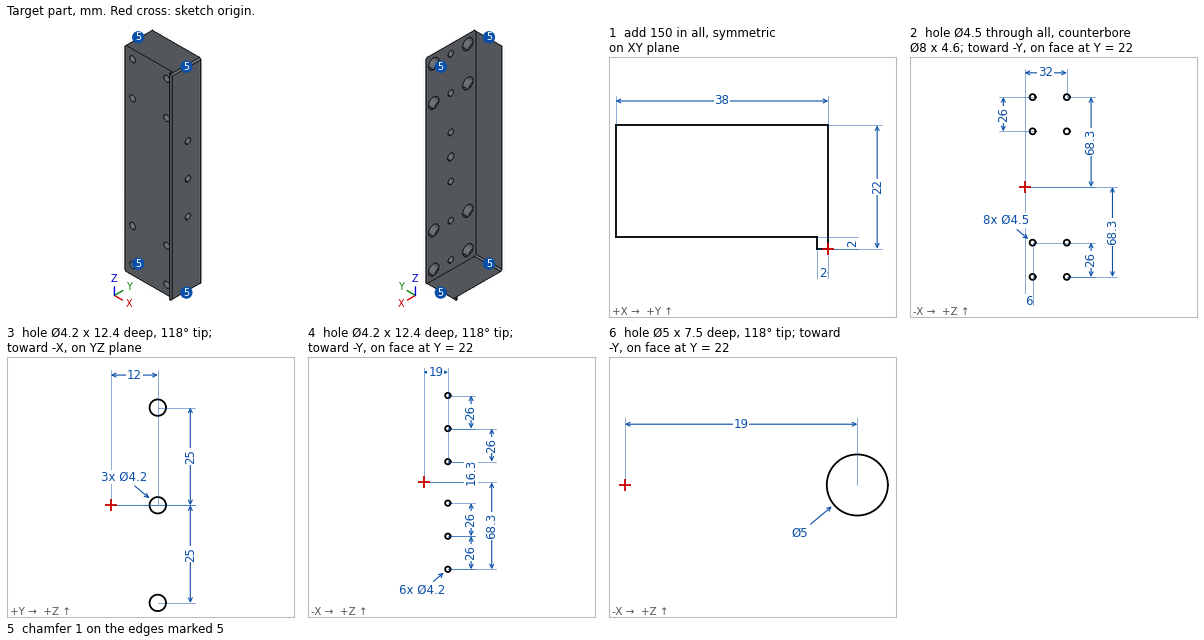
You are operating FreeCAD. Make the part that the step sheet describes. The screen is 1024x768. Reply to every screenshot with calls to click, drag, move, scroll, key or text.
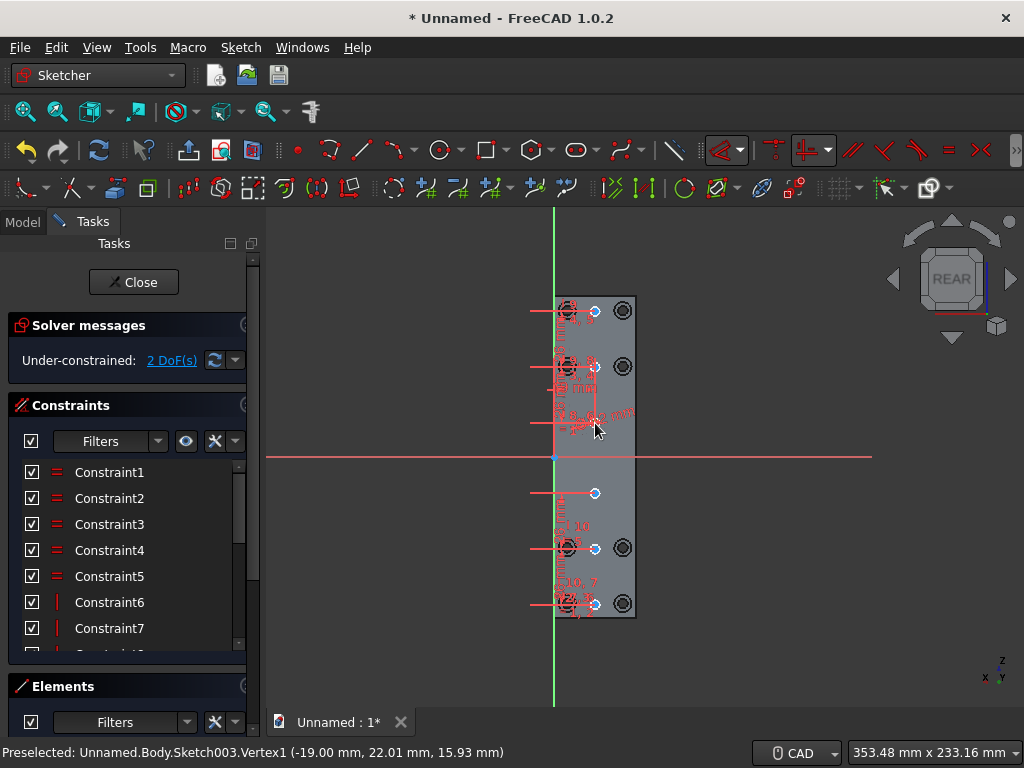
key(i)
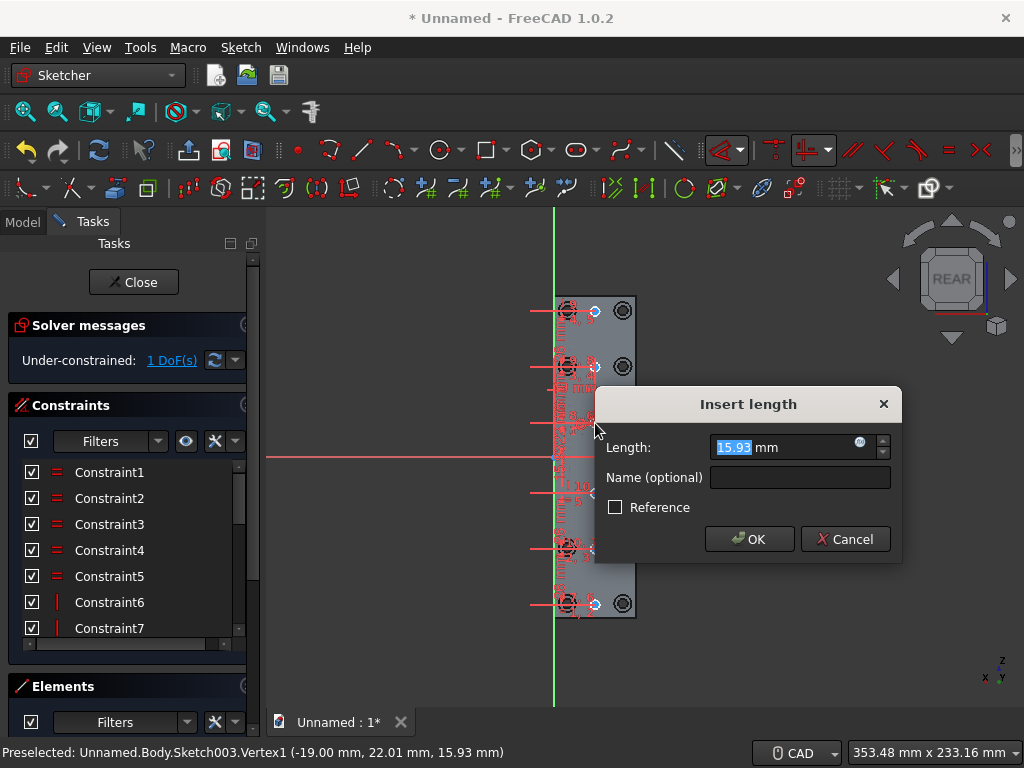
text(16.3)
key(Return)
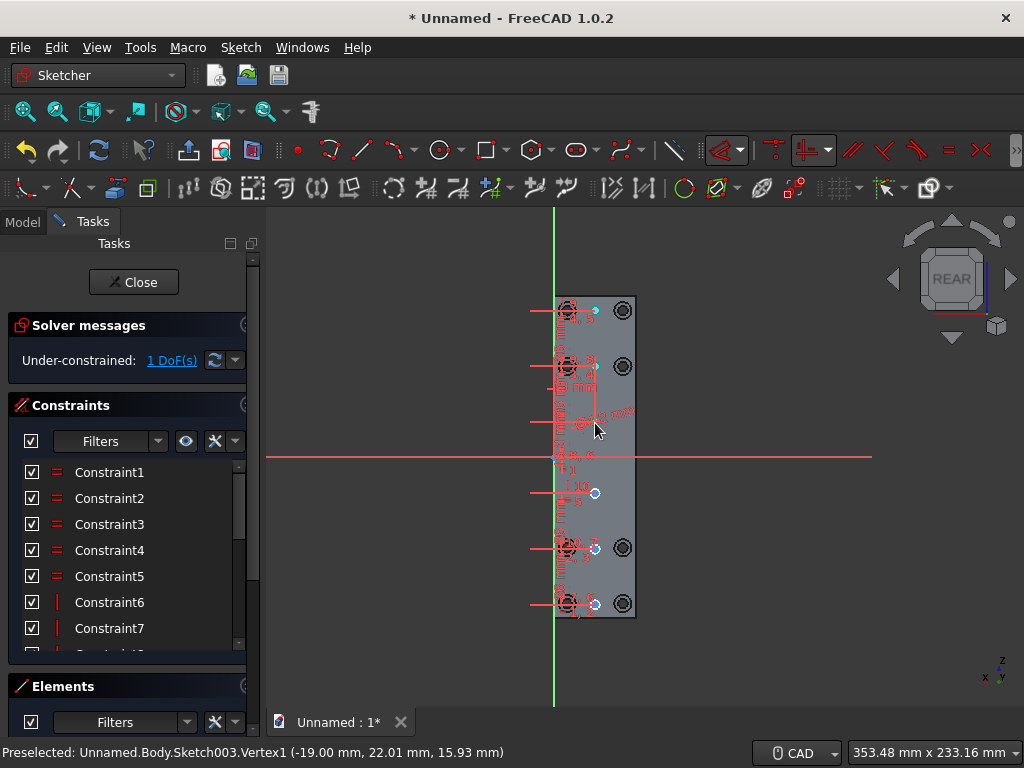
click(595, 605)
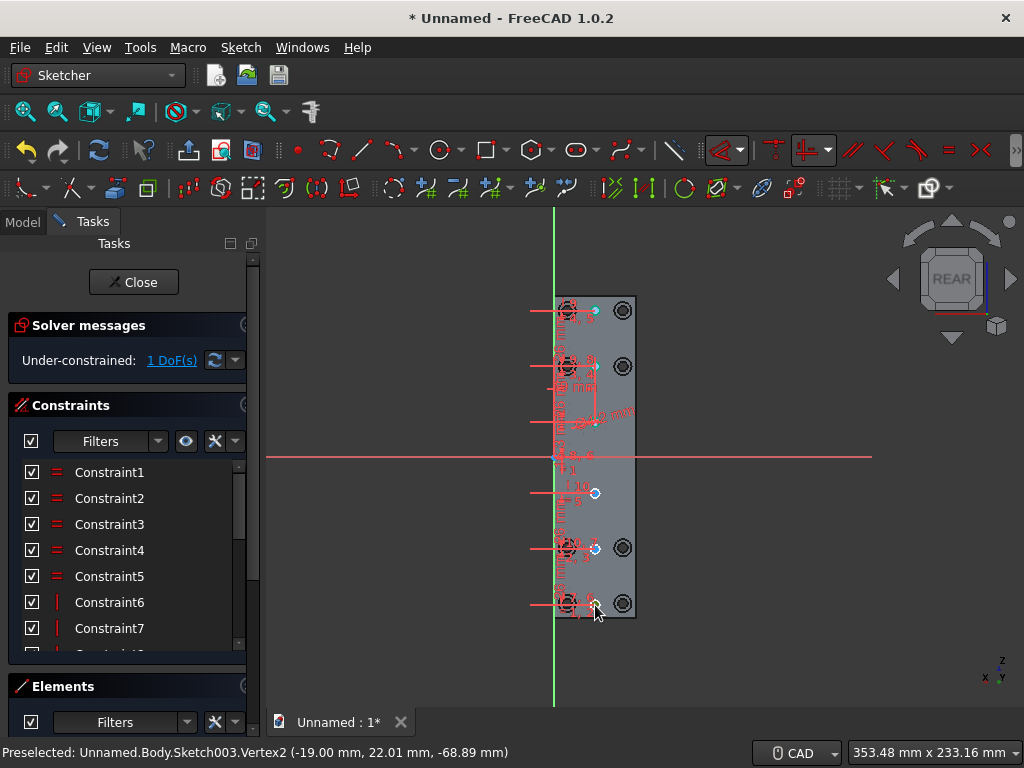
key(i)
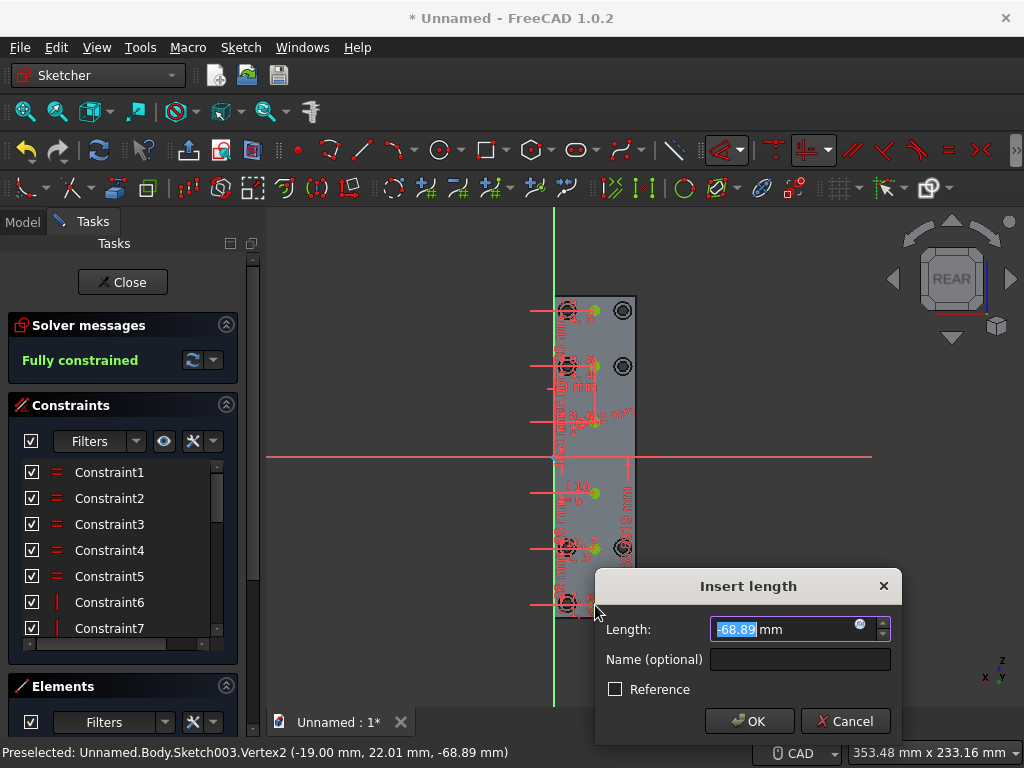
text(-68.3)
key(Return)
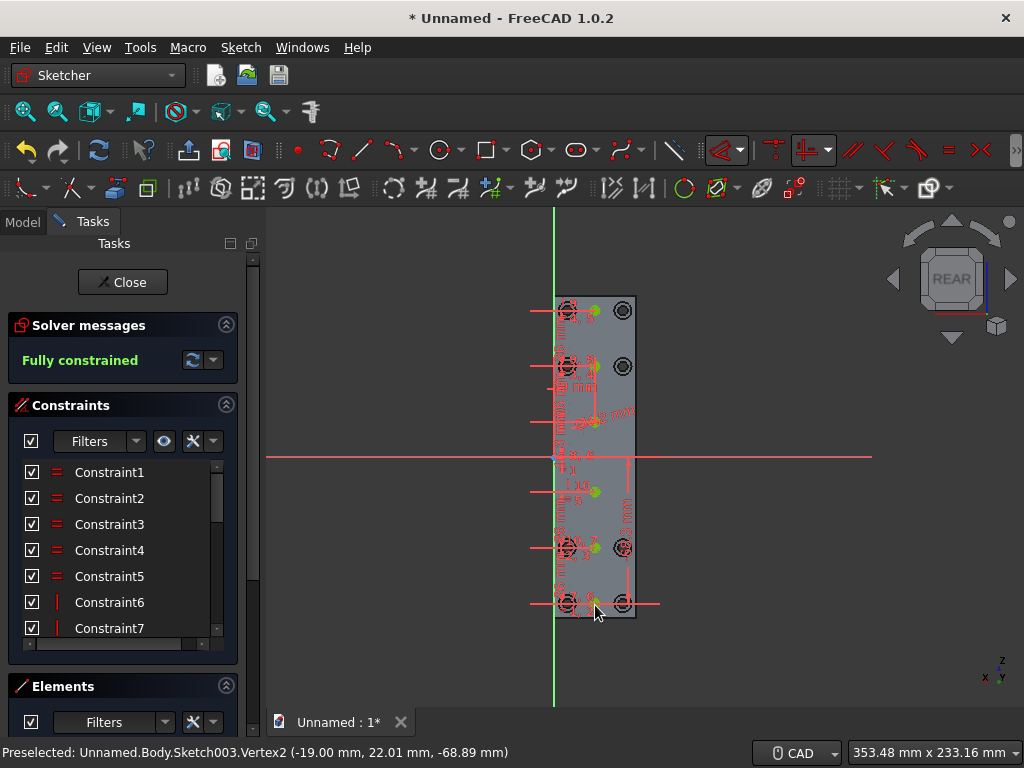
click(123, 282)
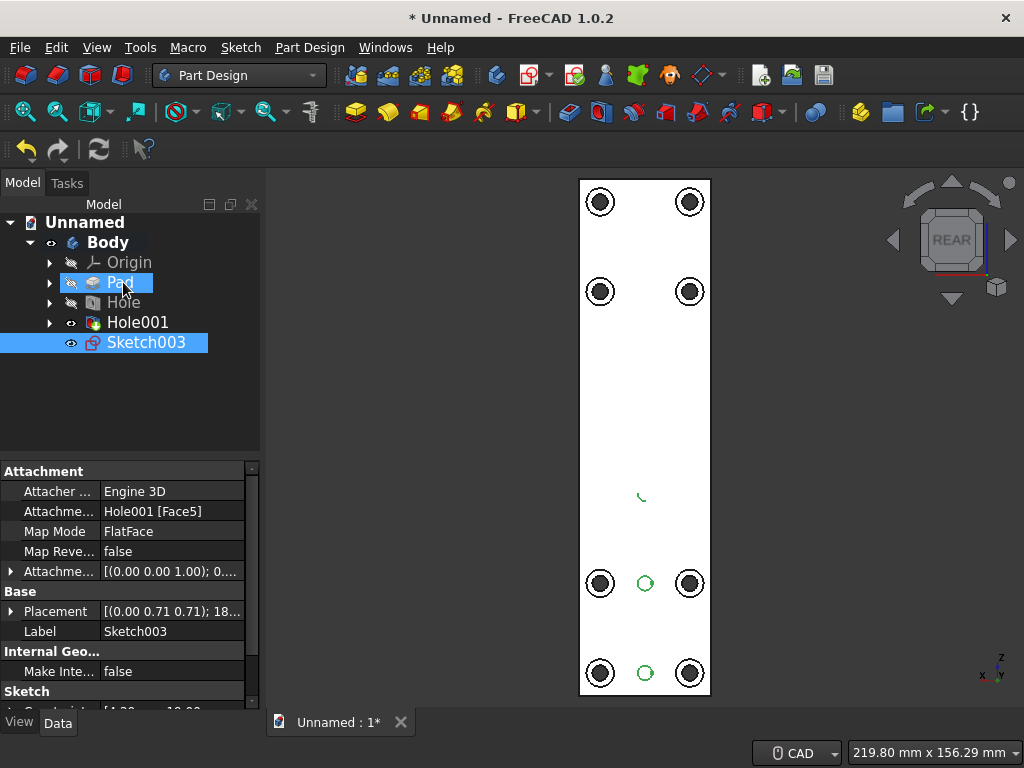
click(602, 112)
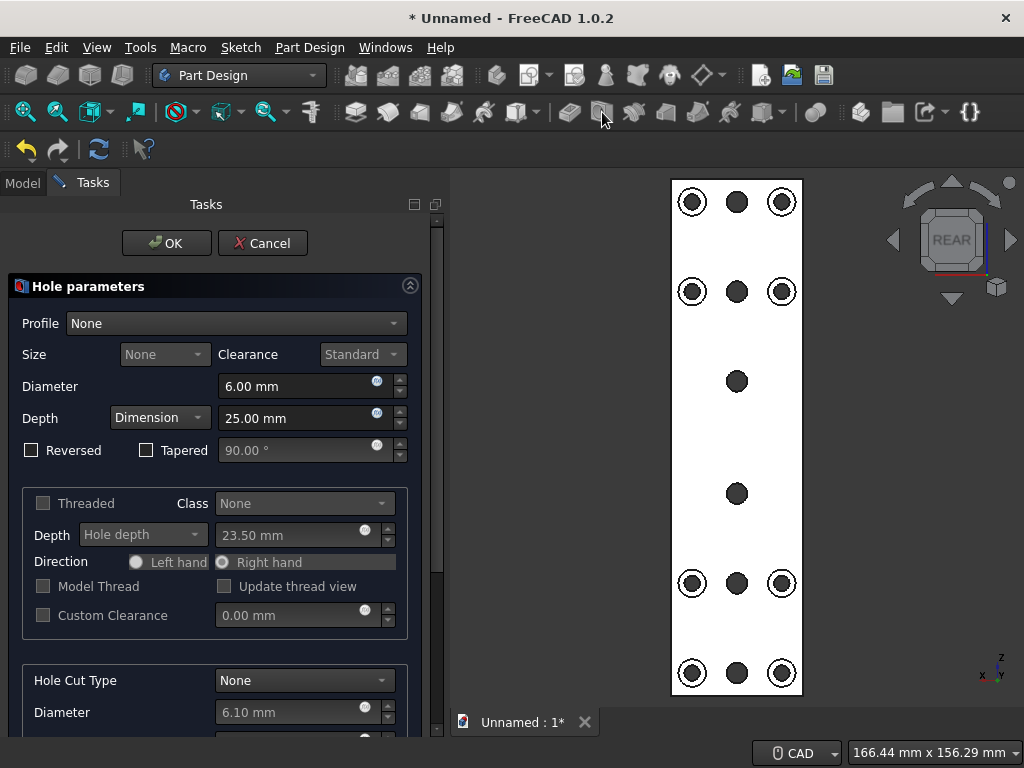
triple_click(305, 386)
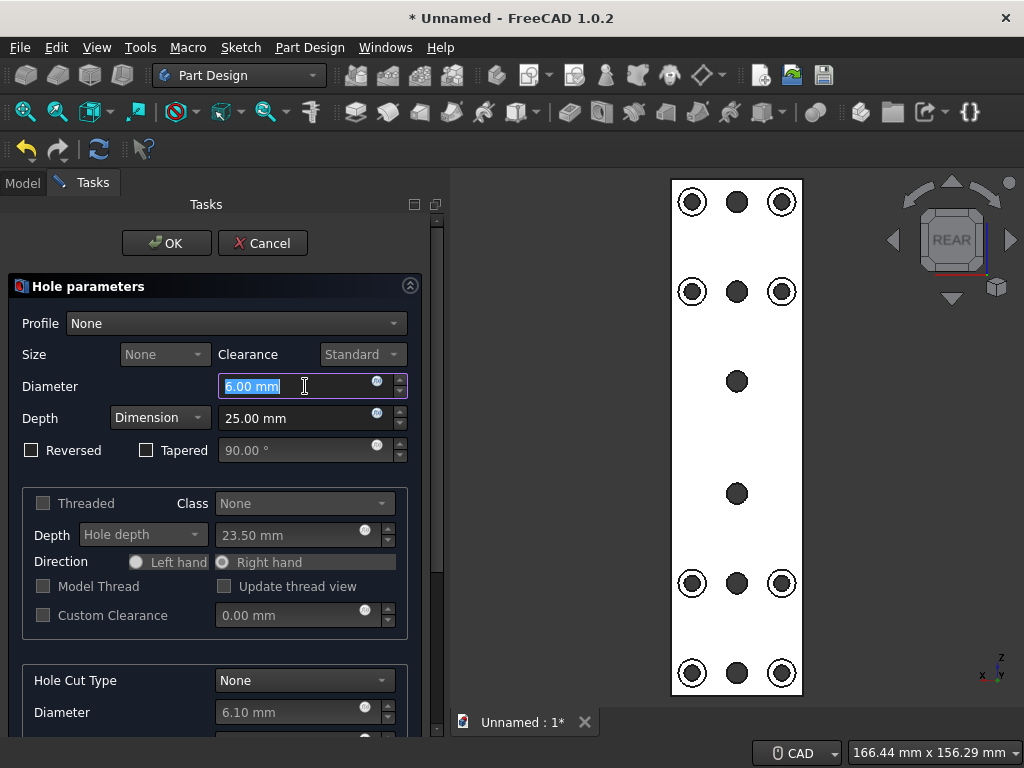
text(4.2)
key(Tab)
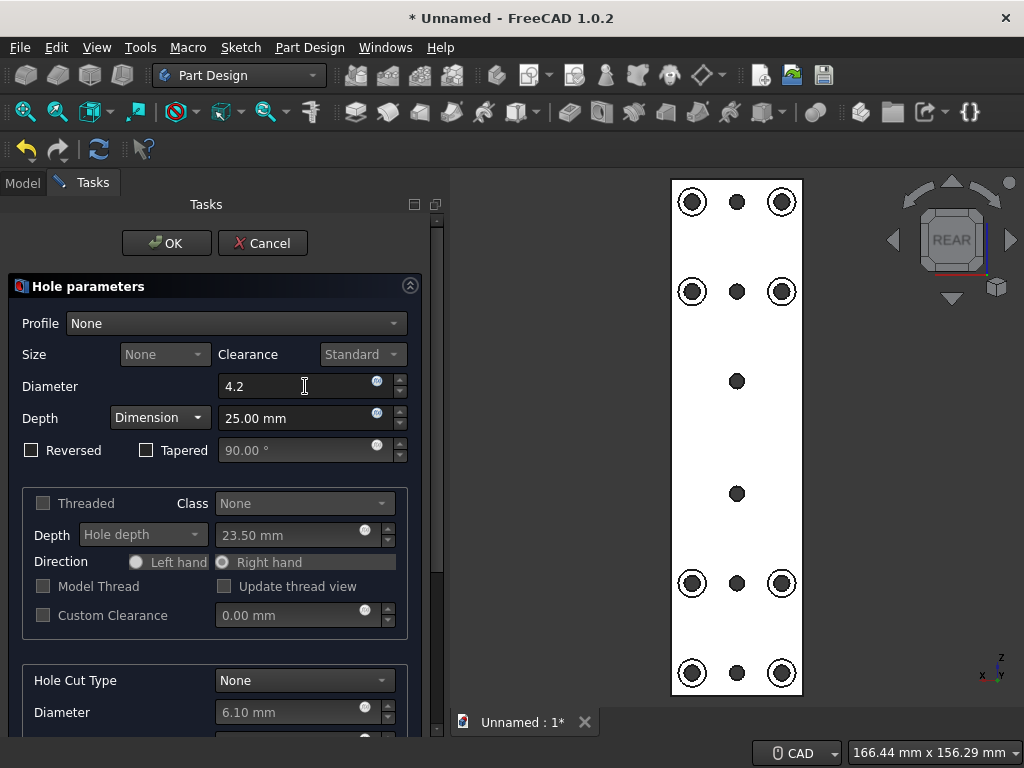
triple_click(305, 418)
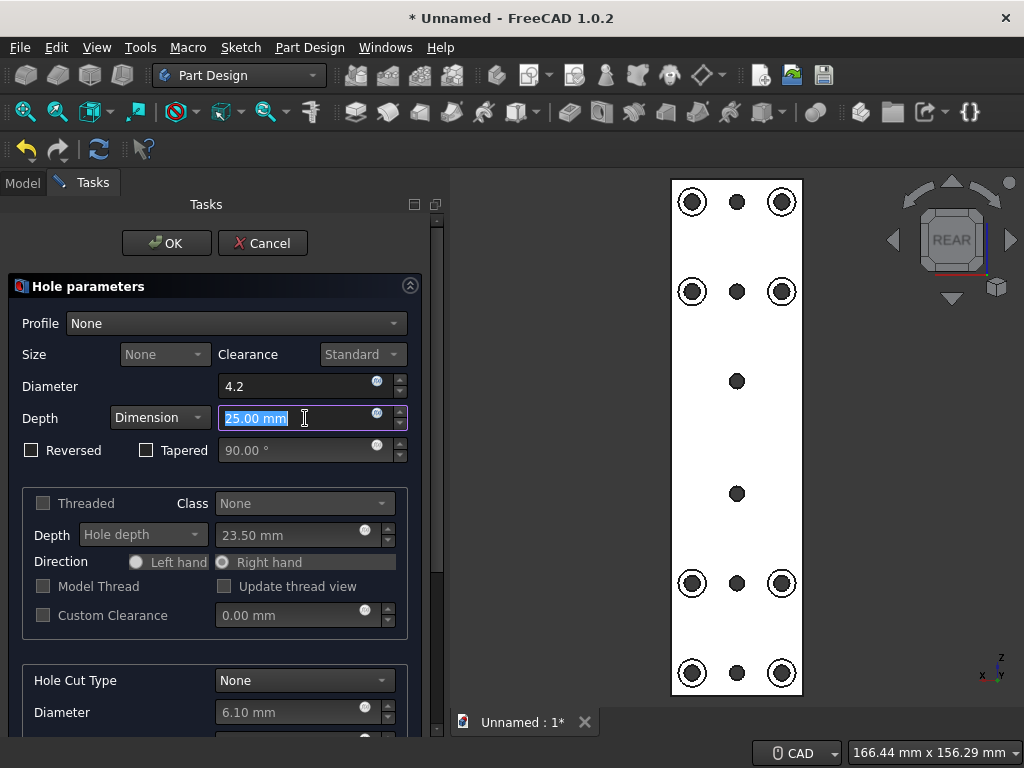
text(12.4)
key(Tab)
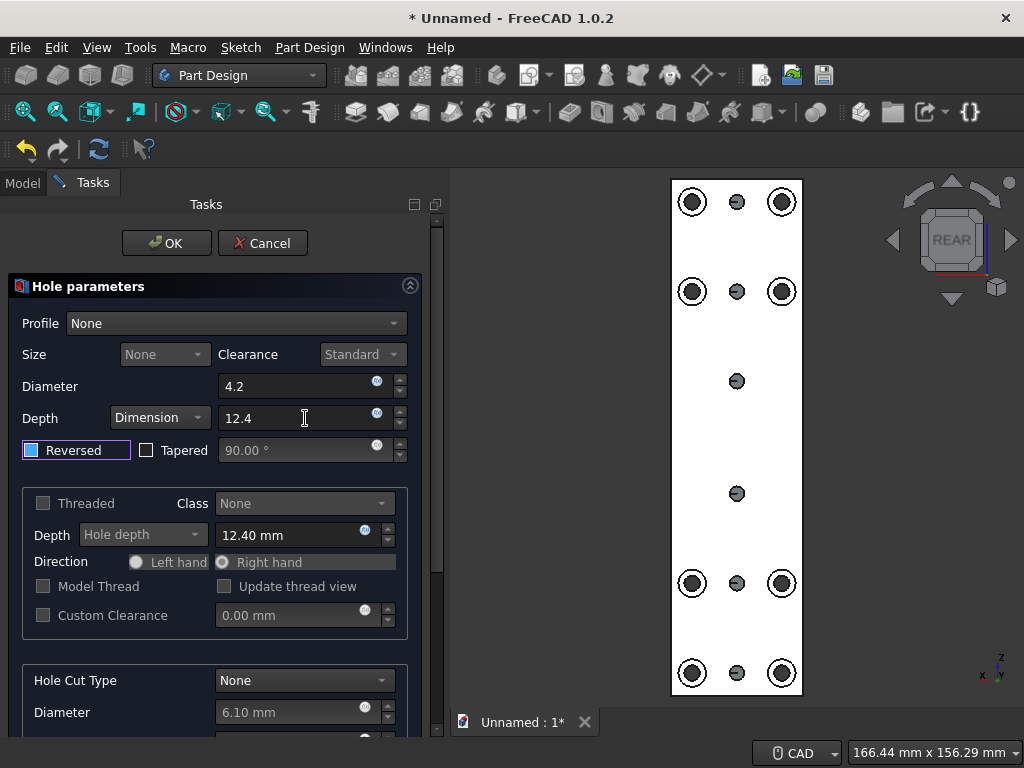
click(167, 243)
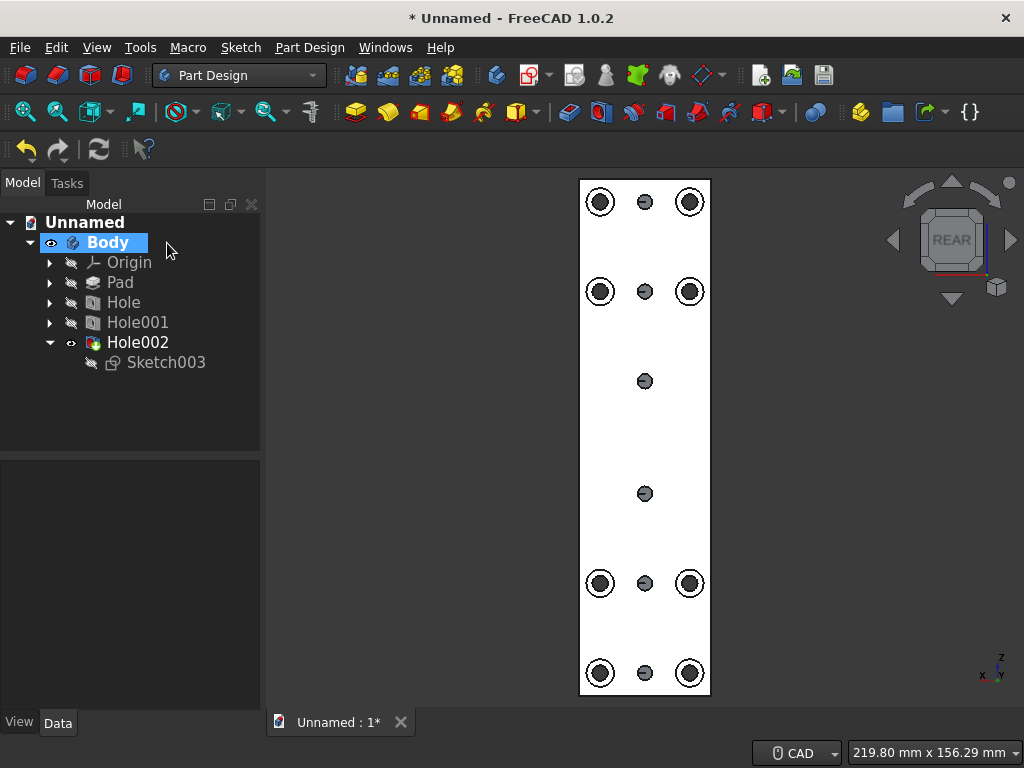
key(0)